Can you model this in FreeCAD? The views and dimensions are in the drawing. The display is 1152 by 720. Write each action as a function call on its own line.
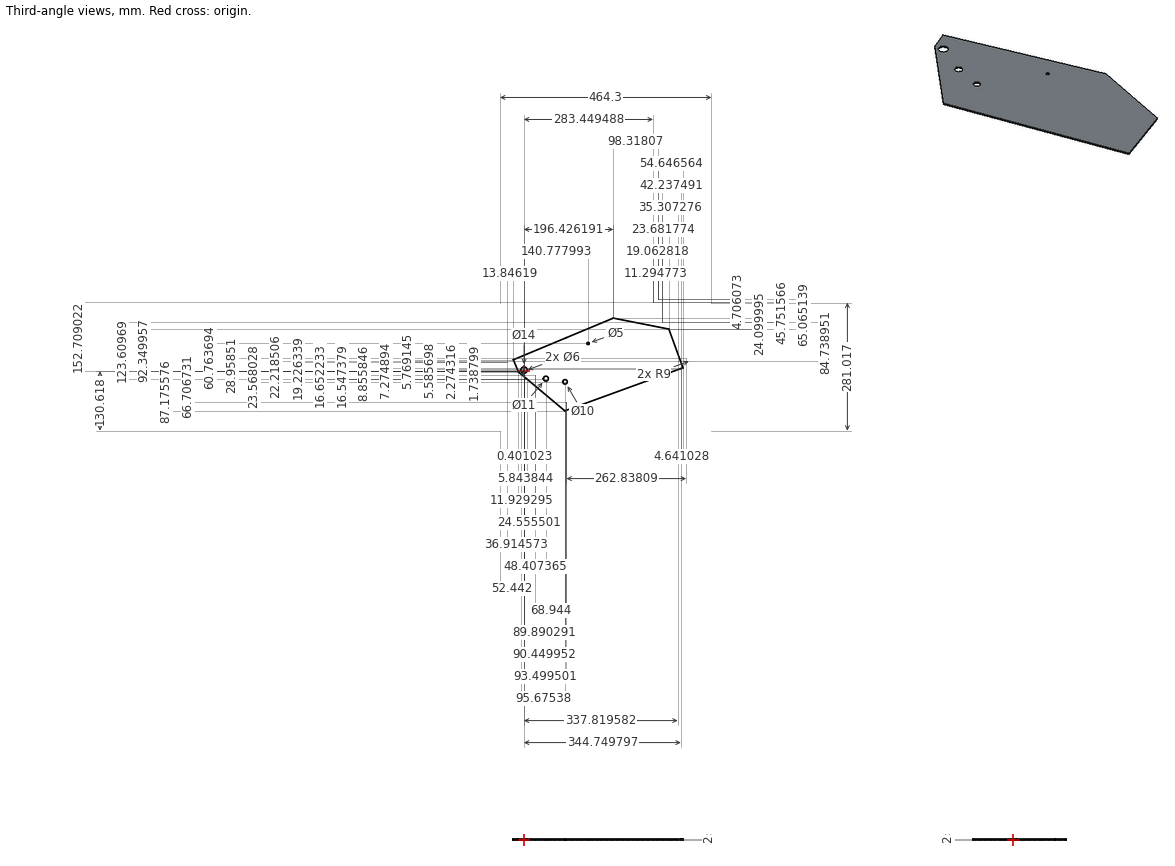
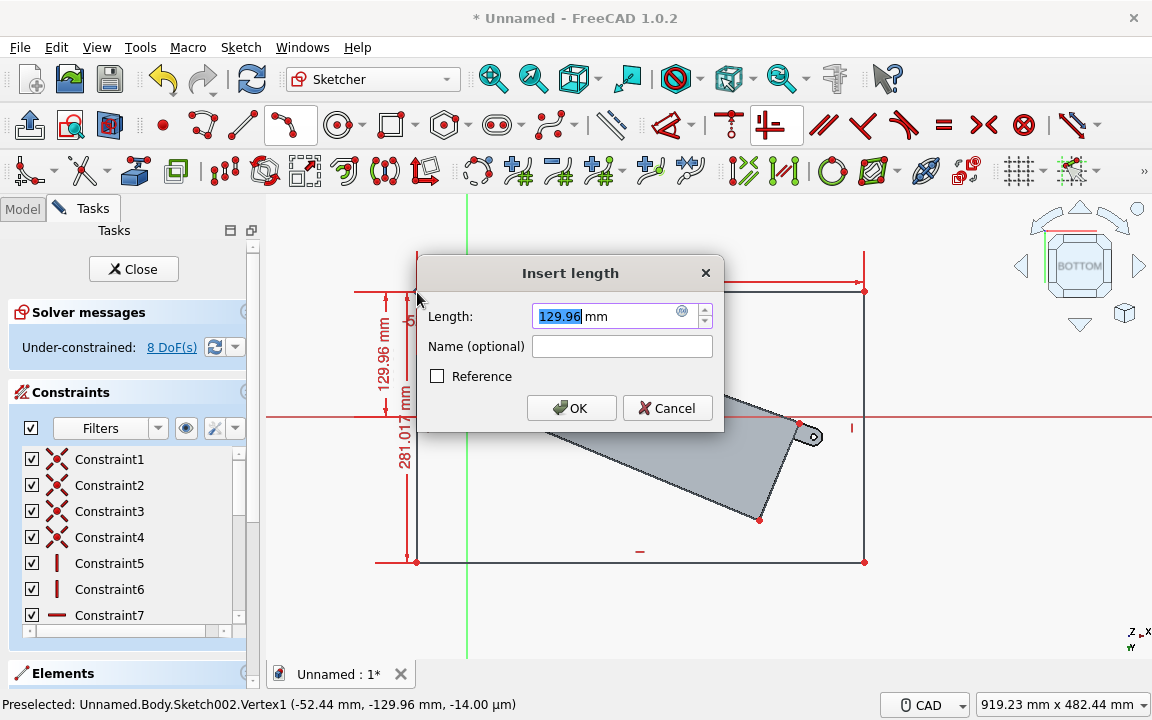
text(130.618)
key(Return)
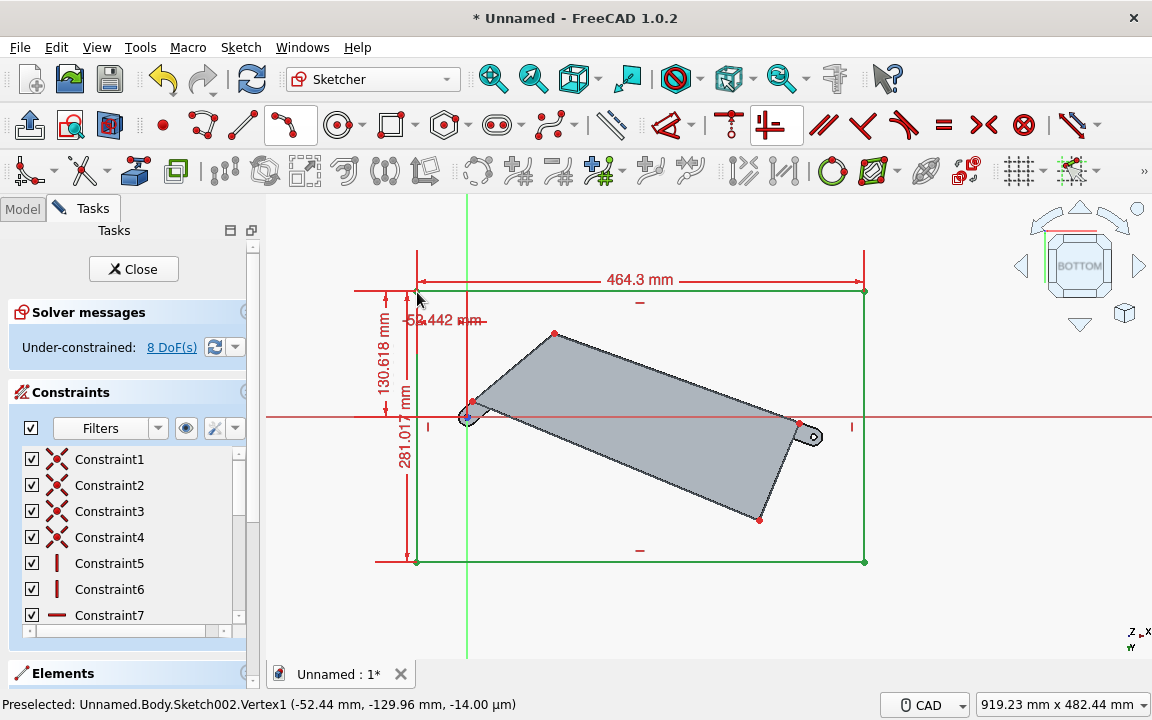
scroll(473, 402, up, 10)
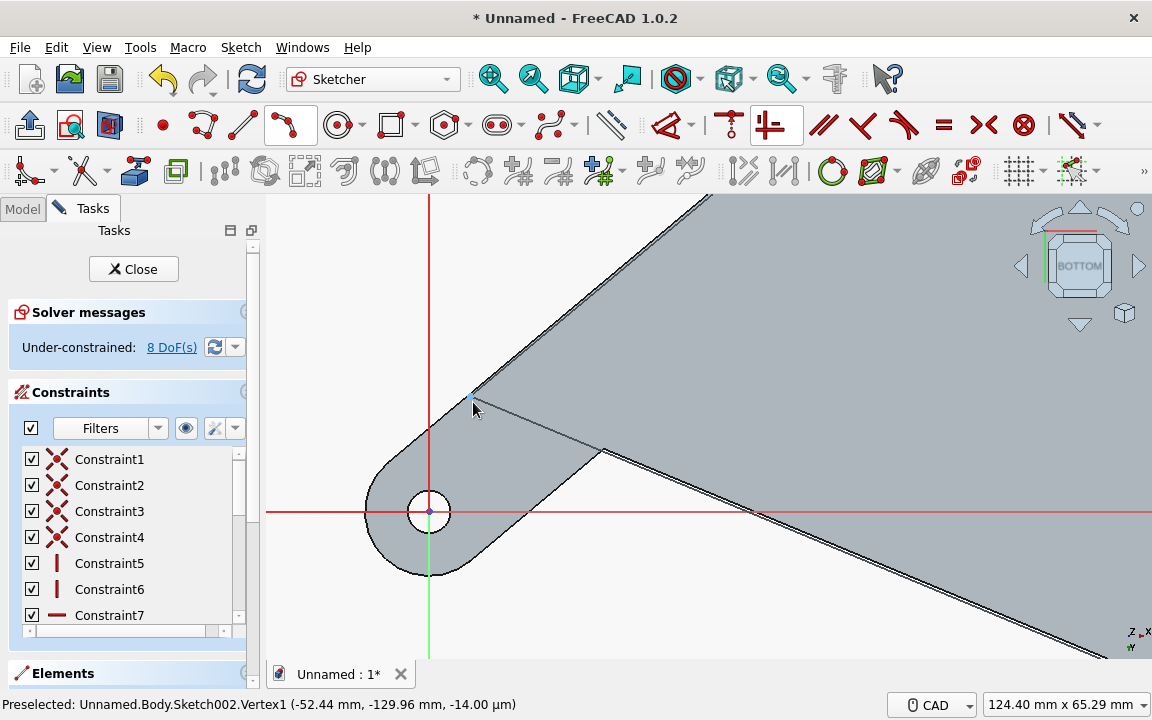
click(470, 396)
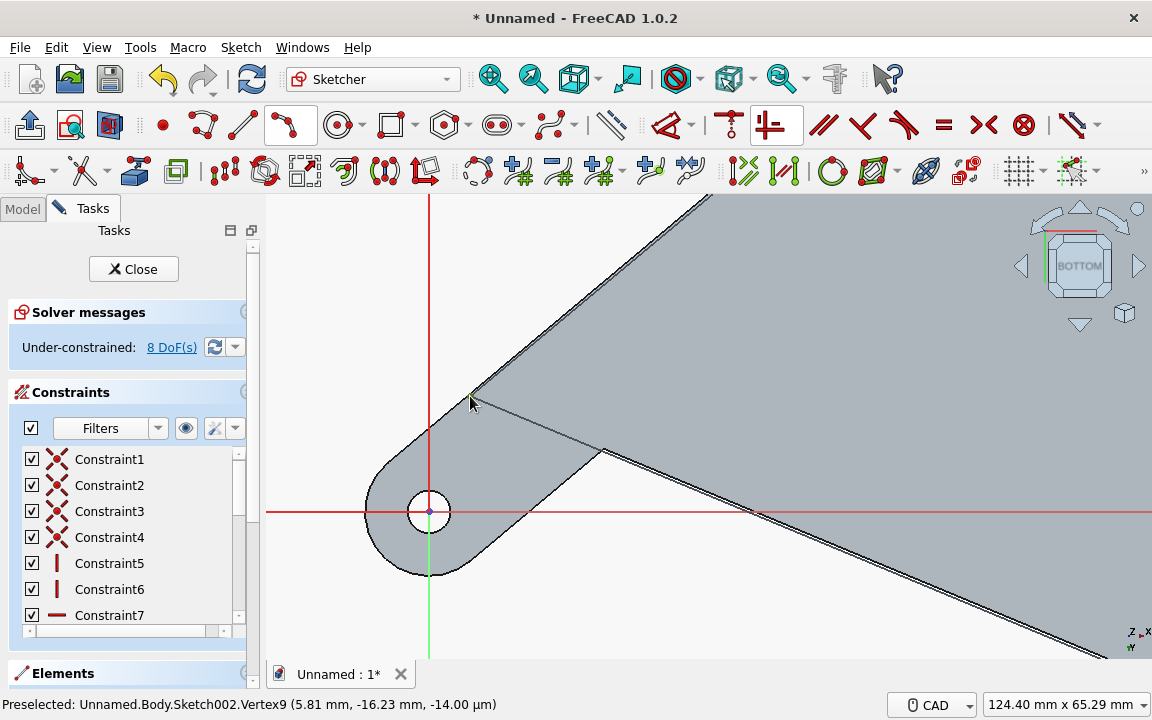
key(l)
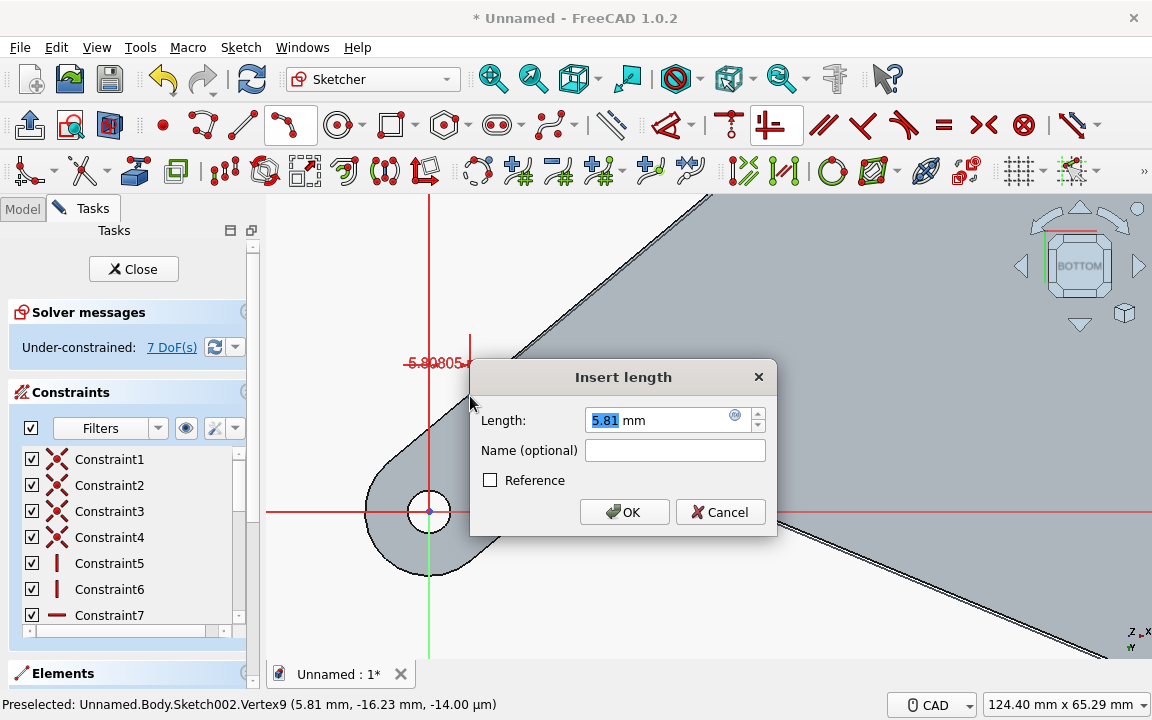
text(5.843844)
key(Return)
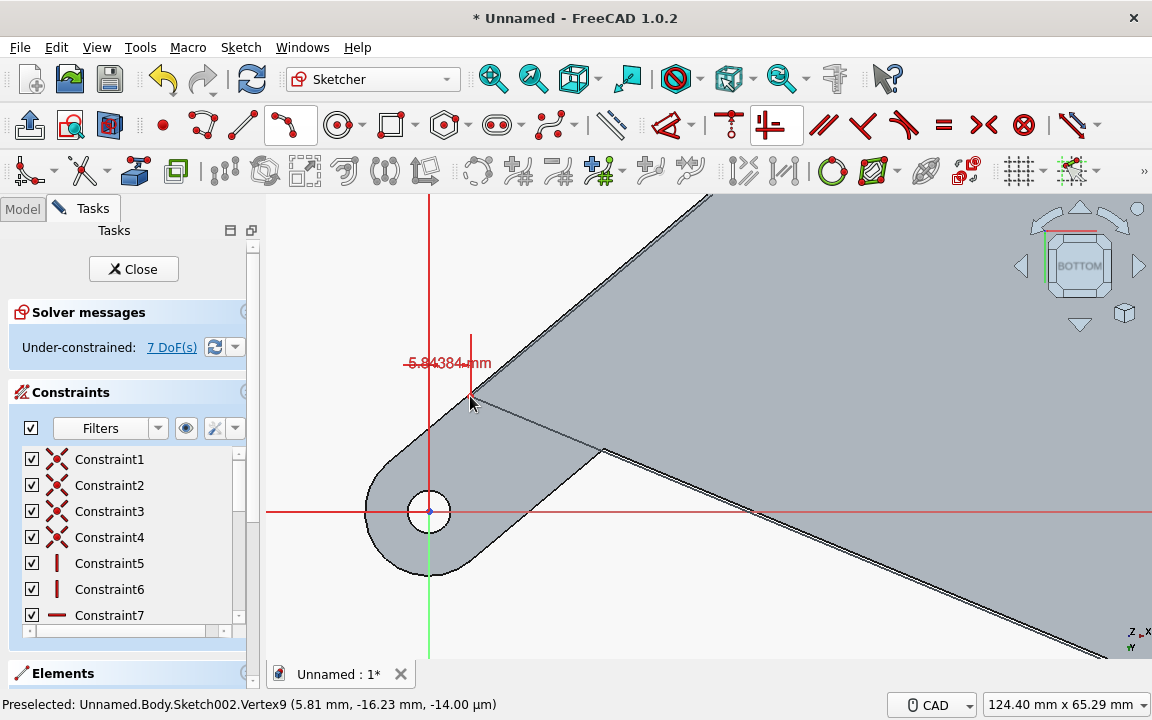
scroll(473, 402, down, 10)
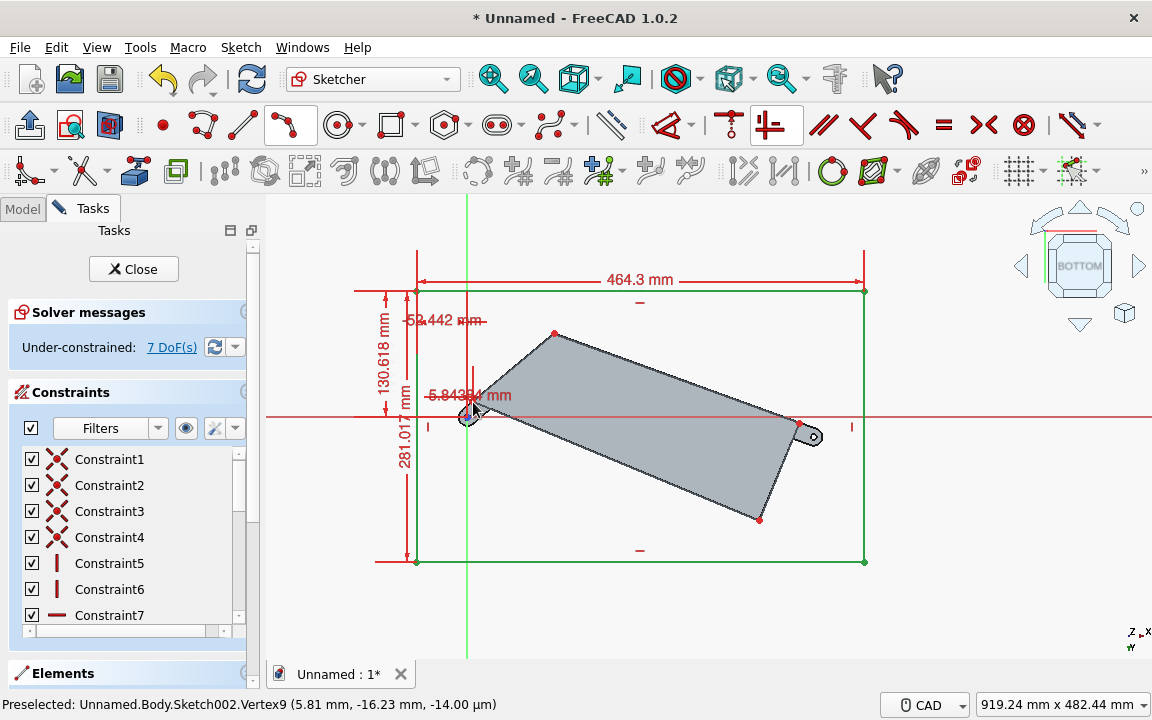
scroll(800, 423, up, 10)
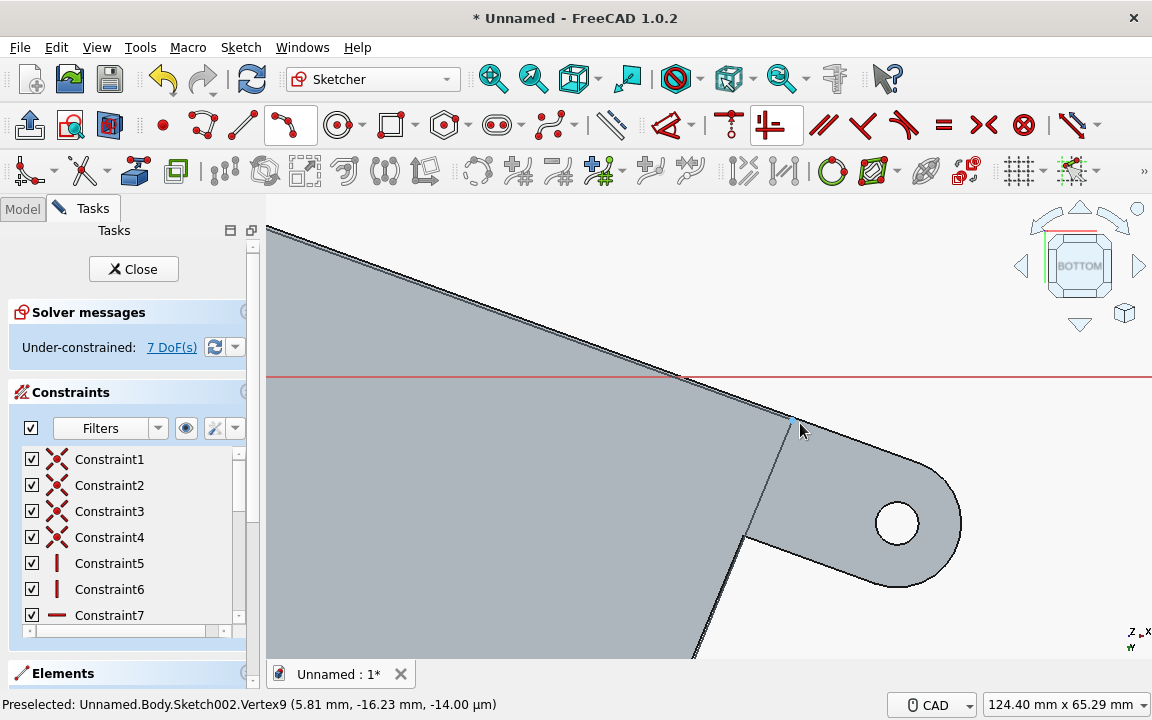
click(793, 420)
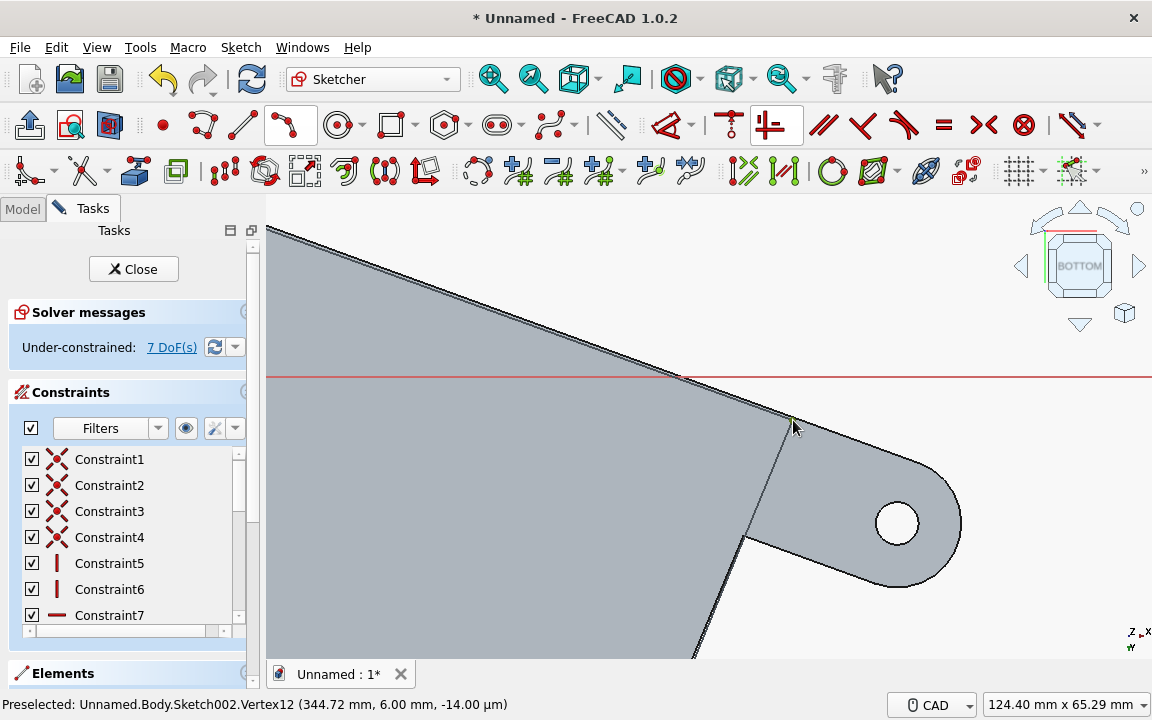
key(i)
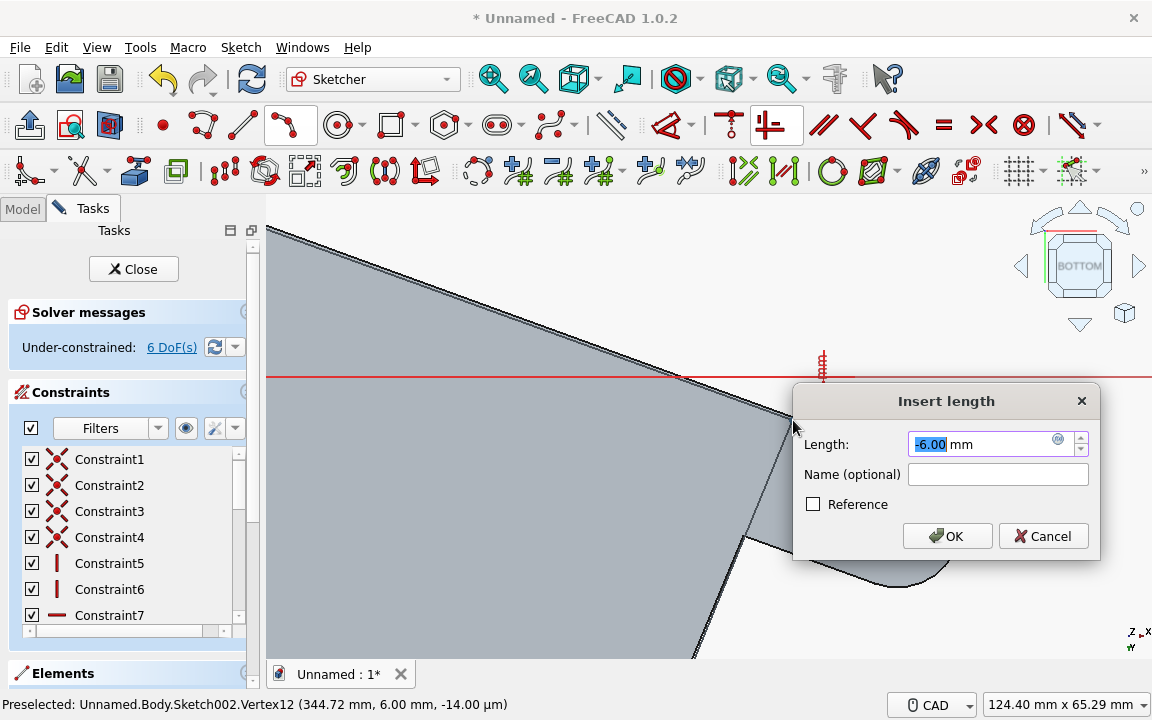
text(-5.585698)
key(Return)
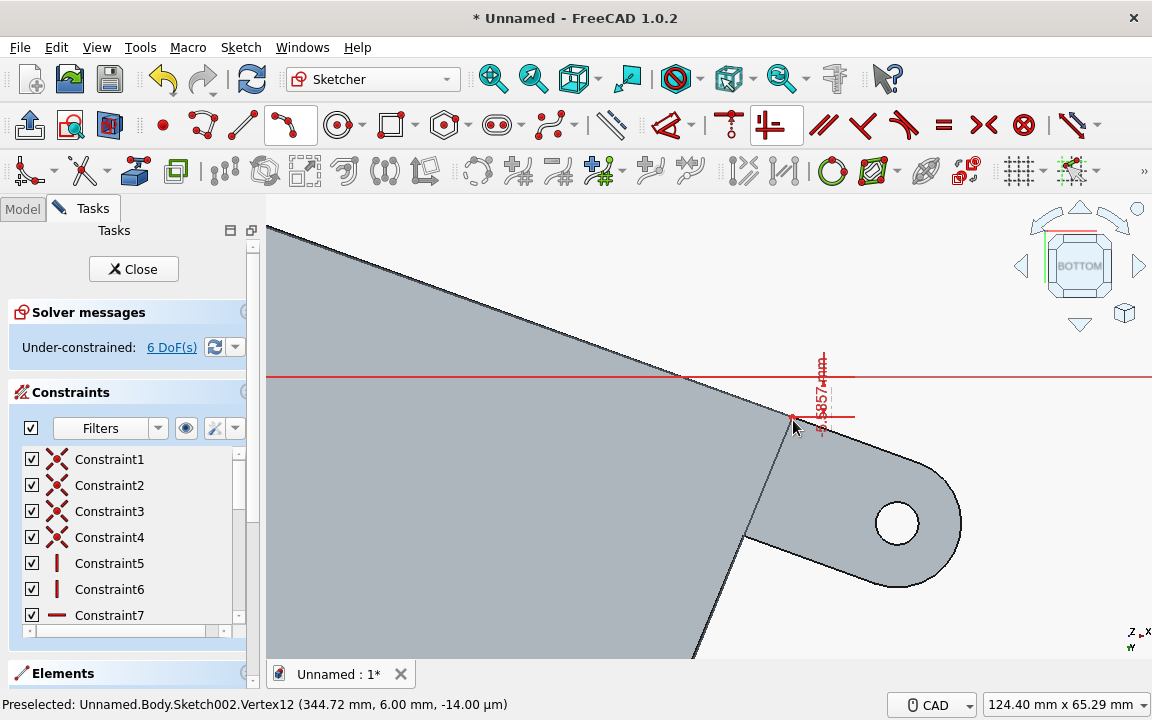
scroll(801, 423, down, 10)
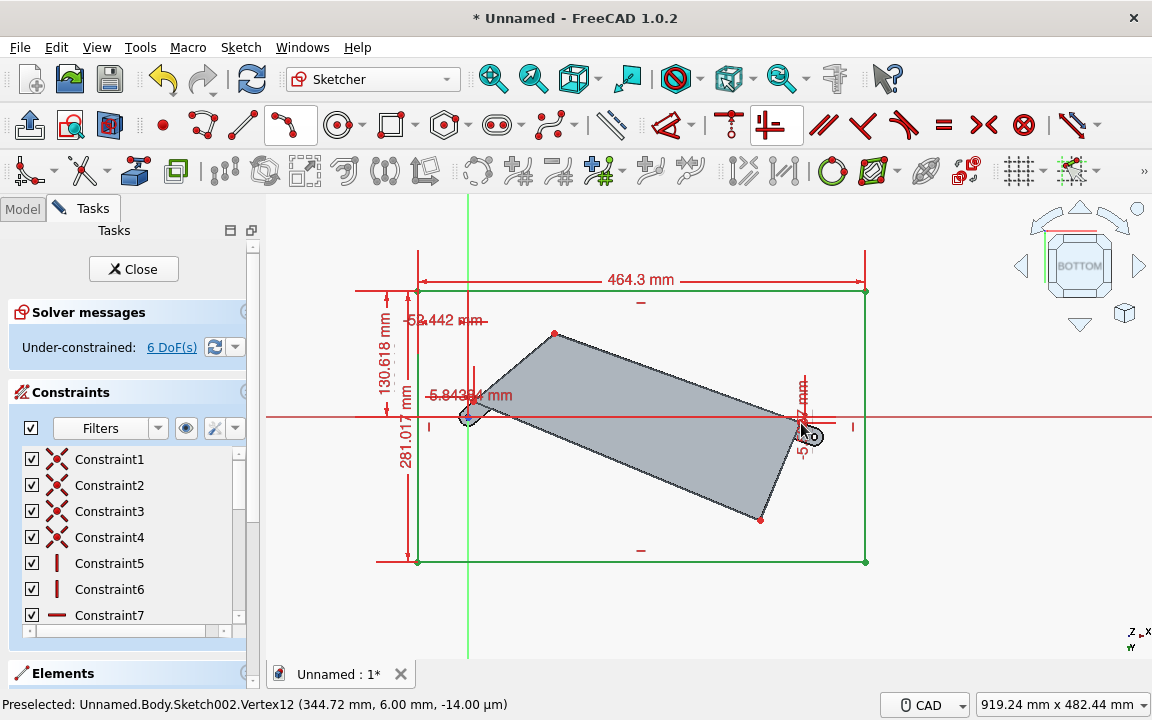
scroll(474, 402, up, 5)